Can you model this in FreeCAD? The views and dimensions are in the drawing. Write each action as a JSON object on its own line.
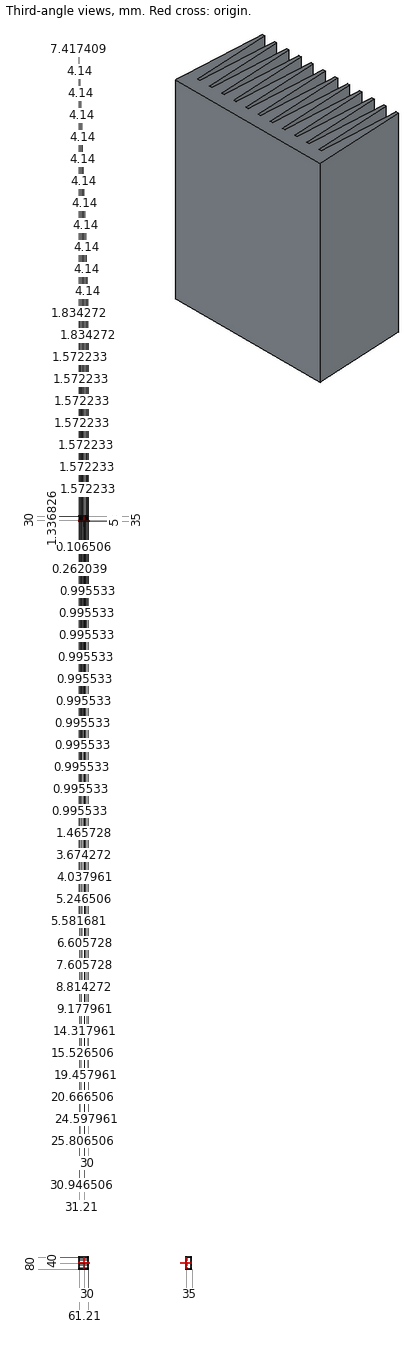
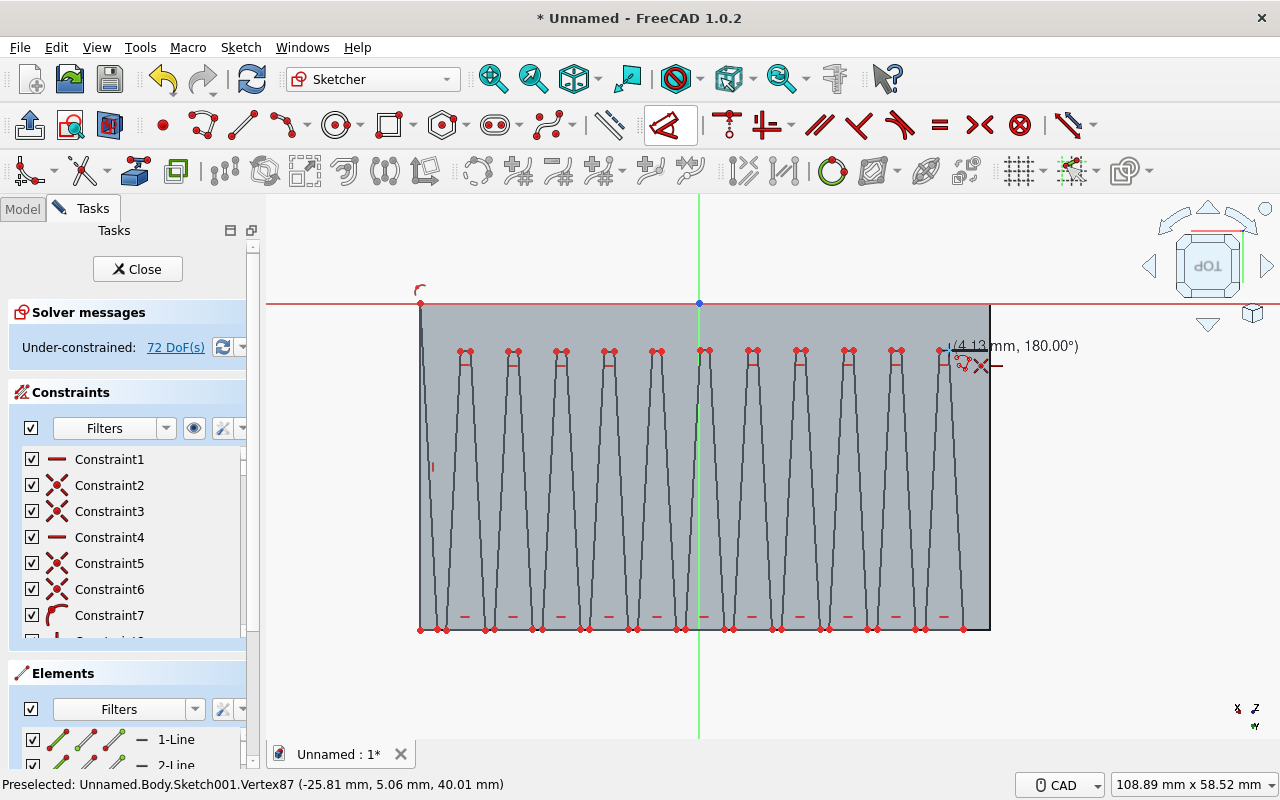
{"action": "scroll", "coordinate": [973, 630], "scroll_direction": "up", "scroll_amount": 3}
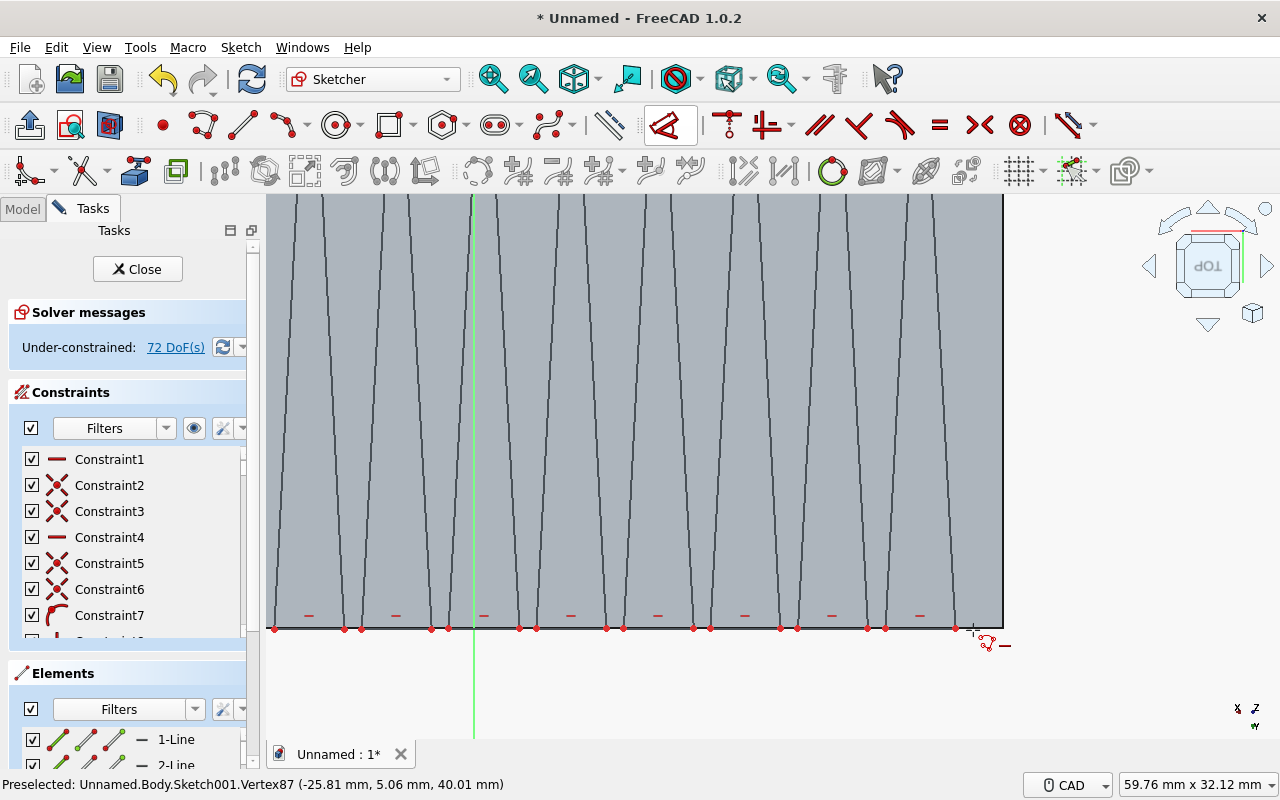
{"action": "left_click", "coordinate": [972, 628]}
{"action": "left_click", "coordinate": [1003, 628]}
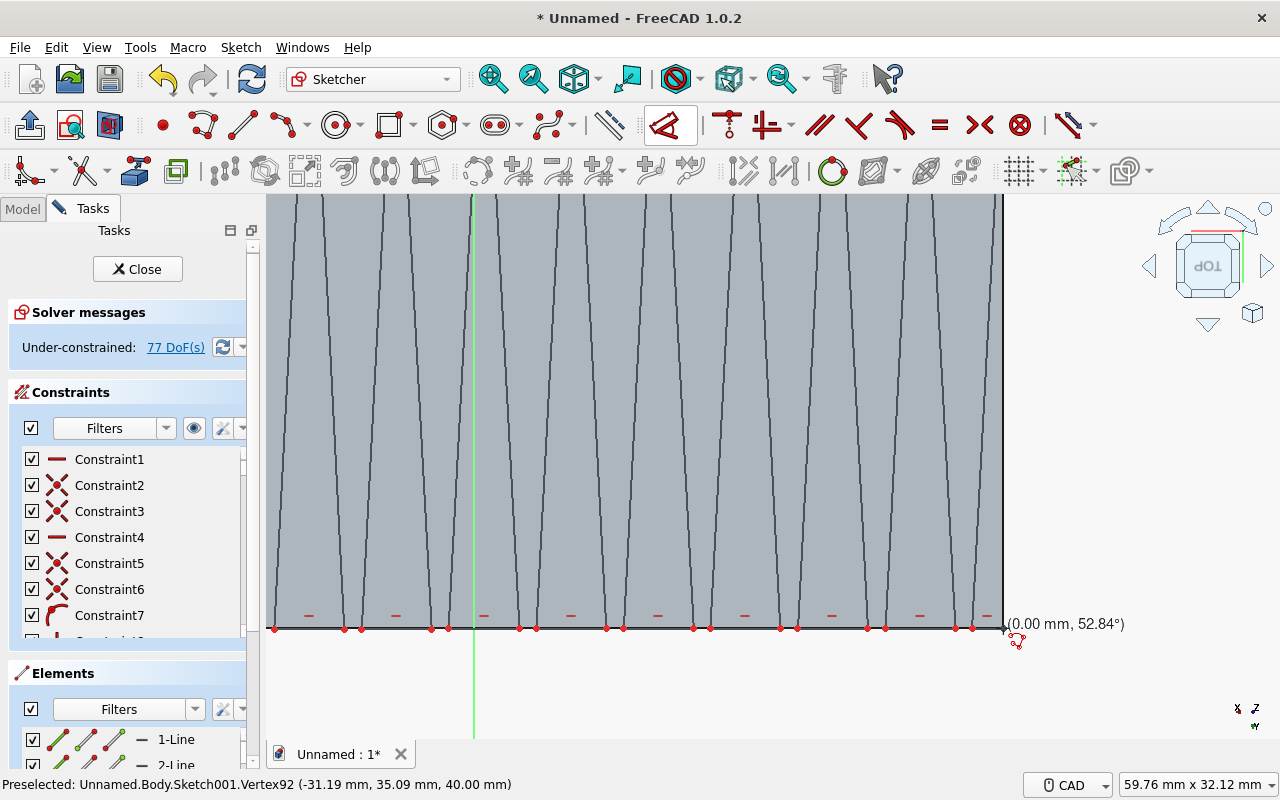
{"action": "scroll", "coordinate": [973, 631], "scroll_direction": "down", "scroll_amount": 3}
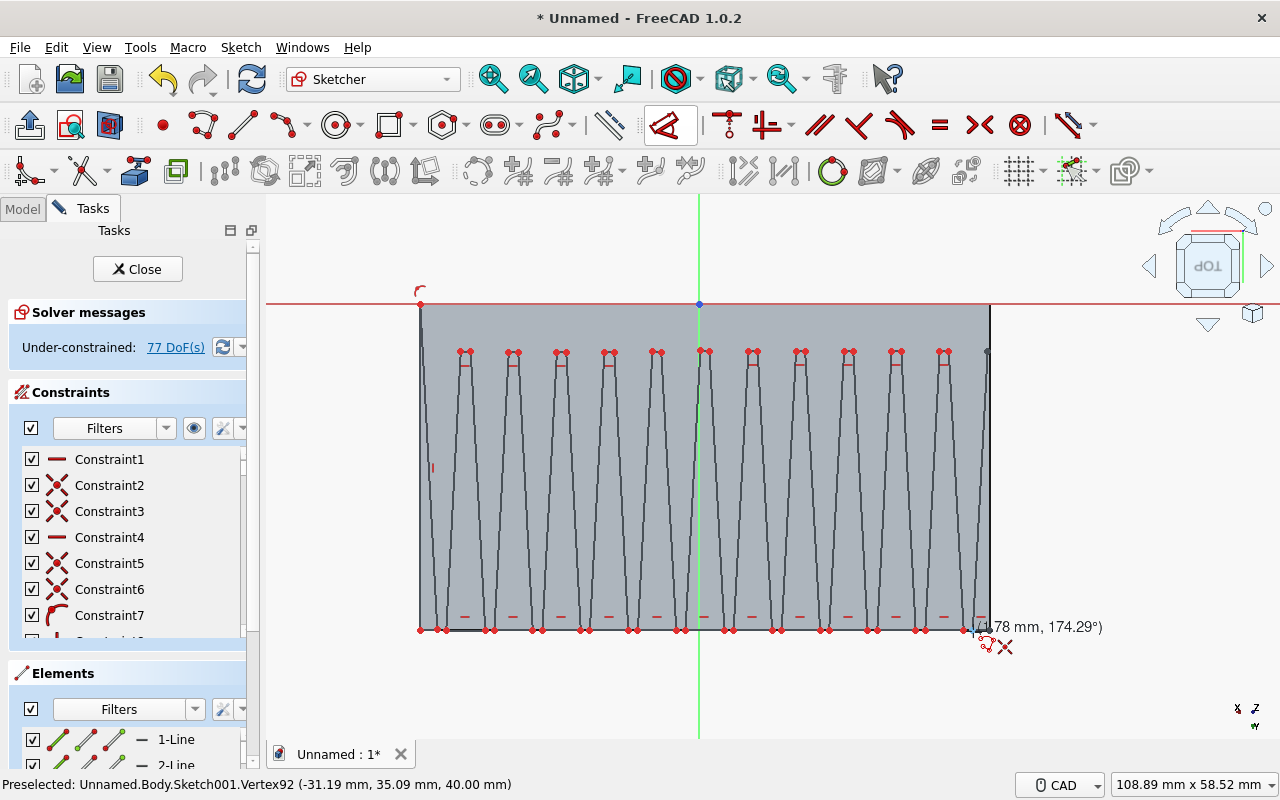
{"action": "scroll", "coordinate": [990, 351], "scroll_direction": "up", "scroll_amount": 10}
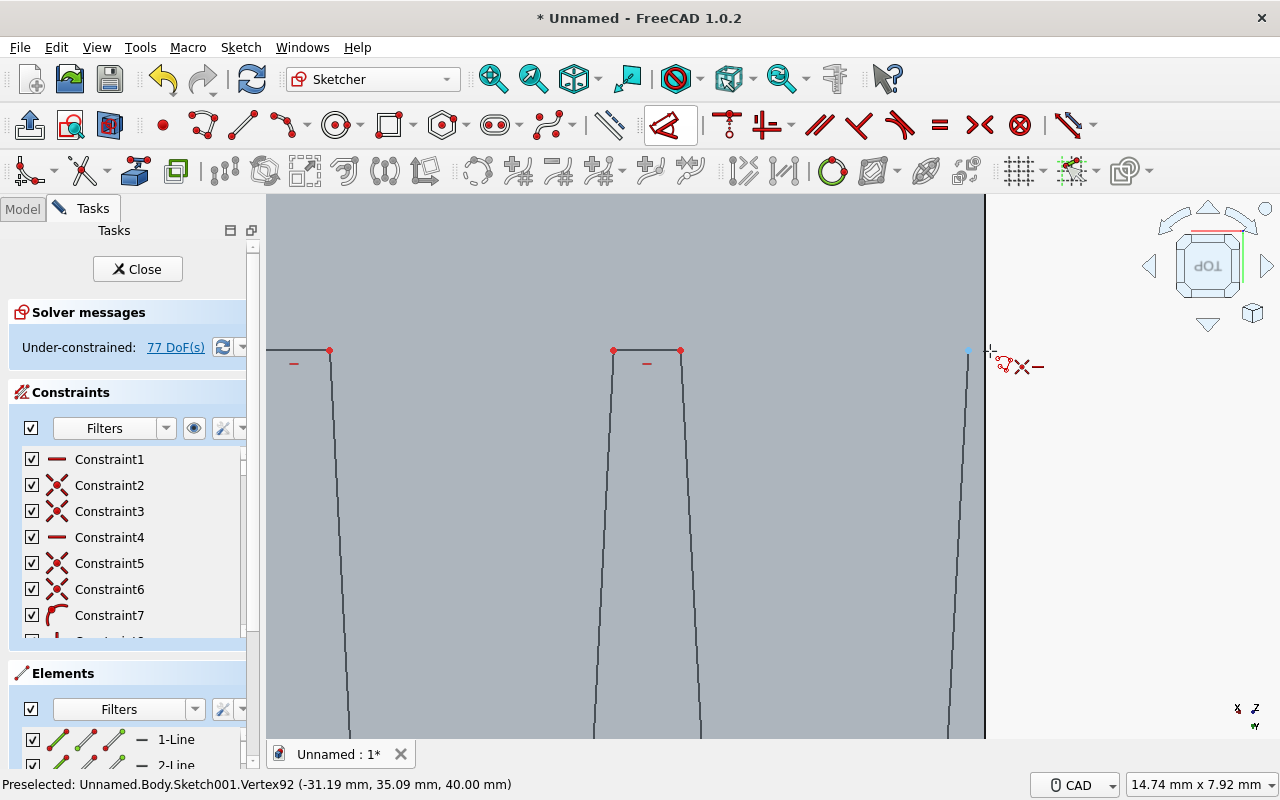
{"action": "left_click", "coordinate": [984, 346]}
{"action": "left_click", "coordinate": [969, 350]}
{"action": "key", "text": "Escape"}
{"action": "key", "text": "Escape"}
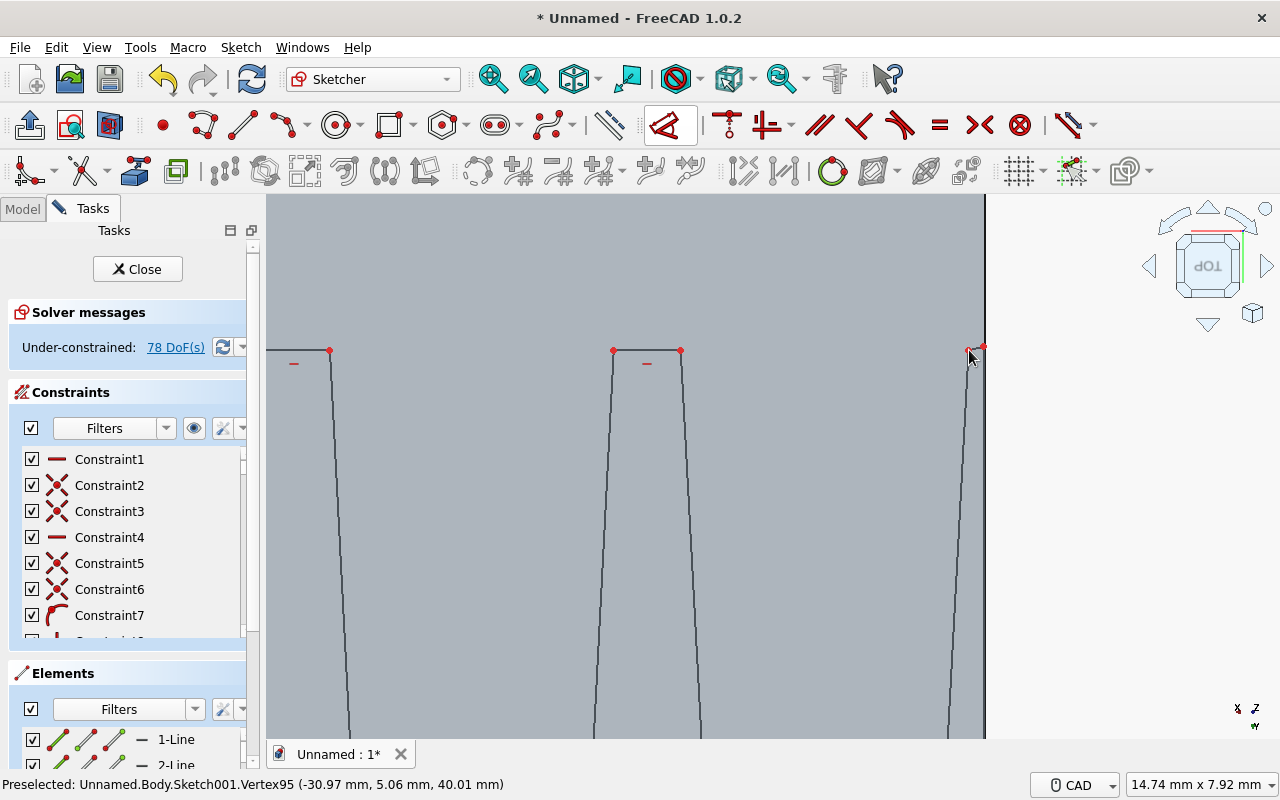
{"action": "scroll", "coordinate": [990, 351], "scroll_direction": "down", "scroll_amount": 10}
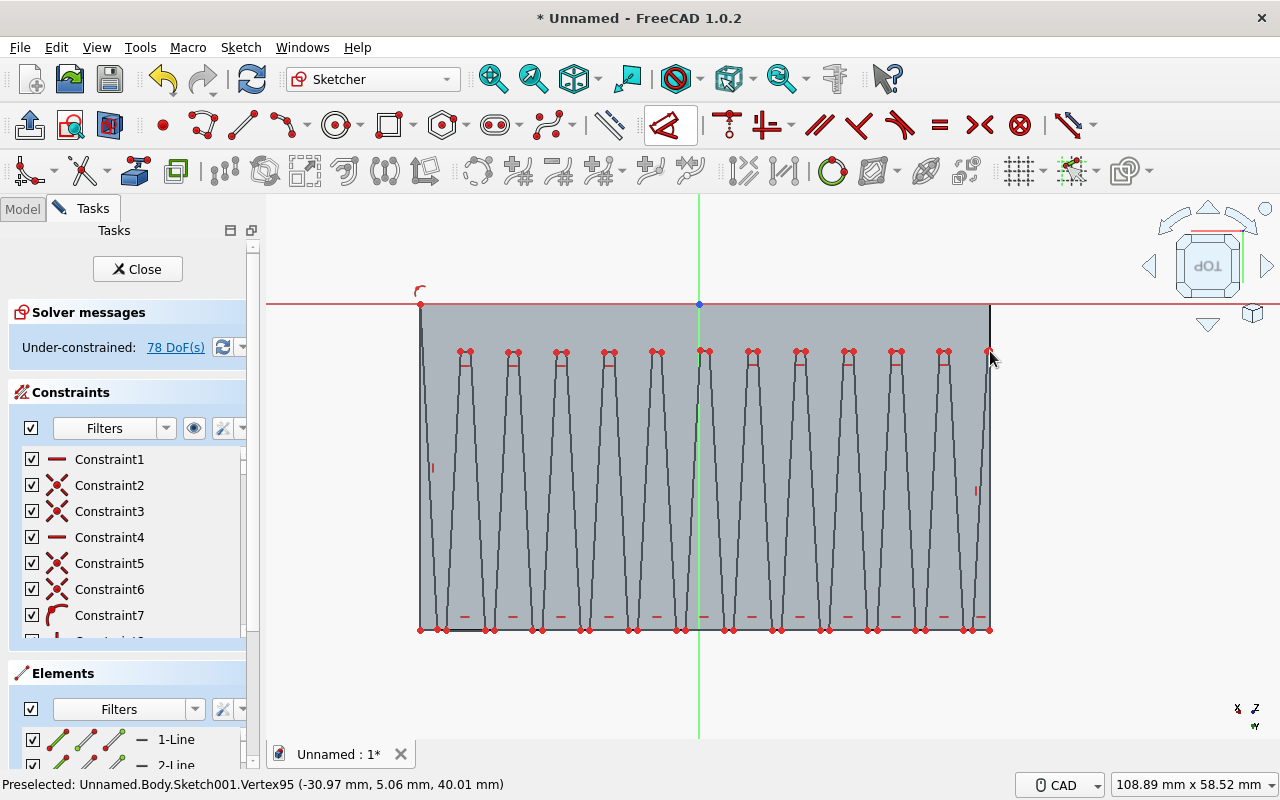
{"action": "scroll", "coordinate": [425, 630], "scroll_direction": "up", "scroll_amount": 5}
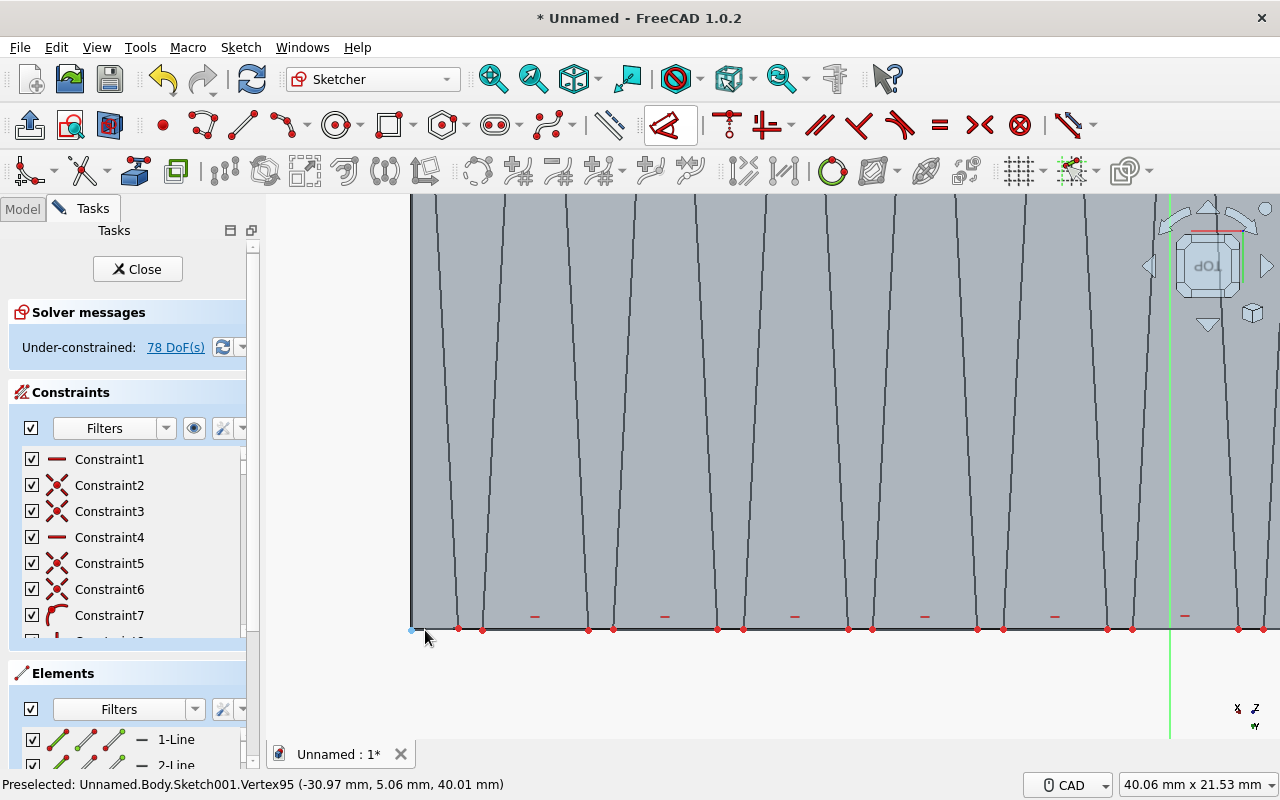
{"action": "left_click", "coordinate": [426, 630]}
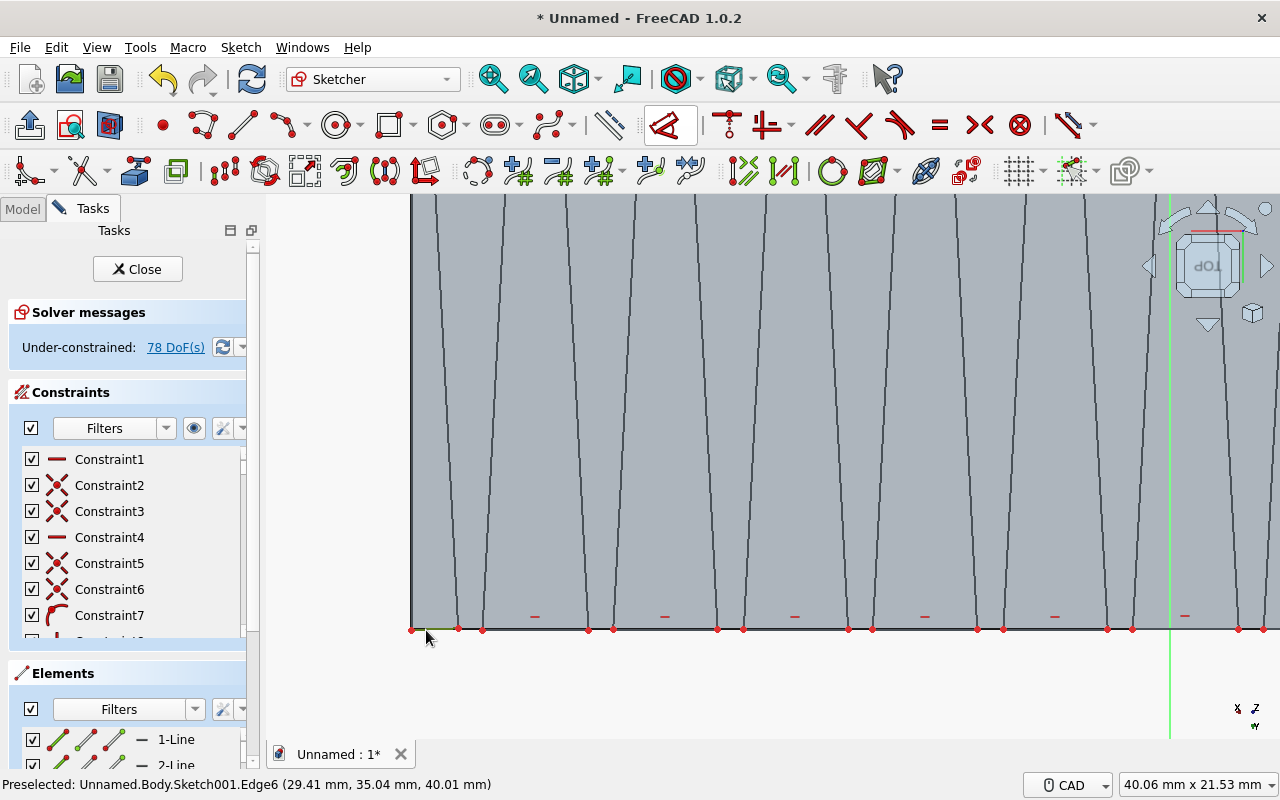
{"action": "left_click", "coordinate": [794, 126]}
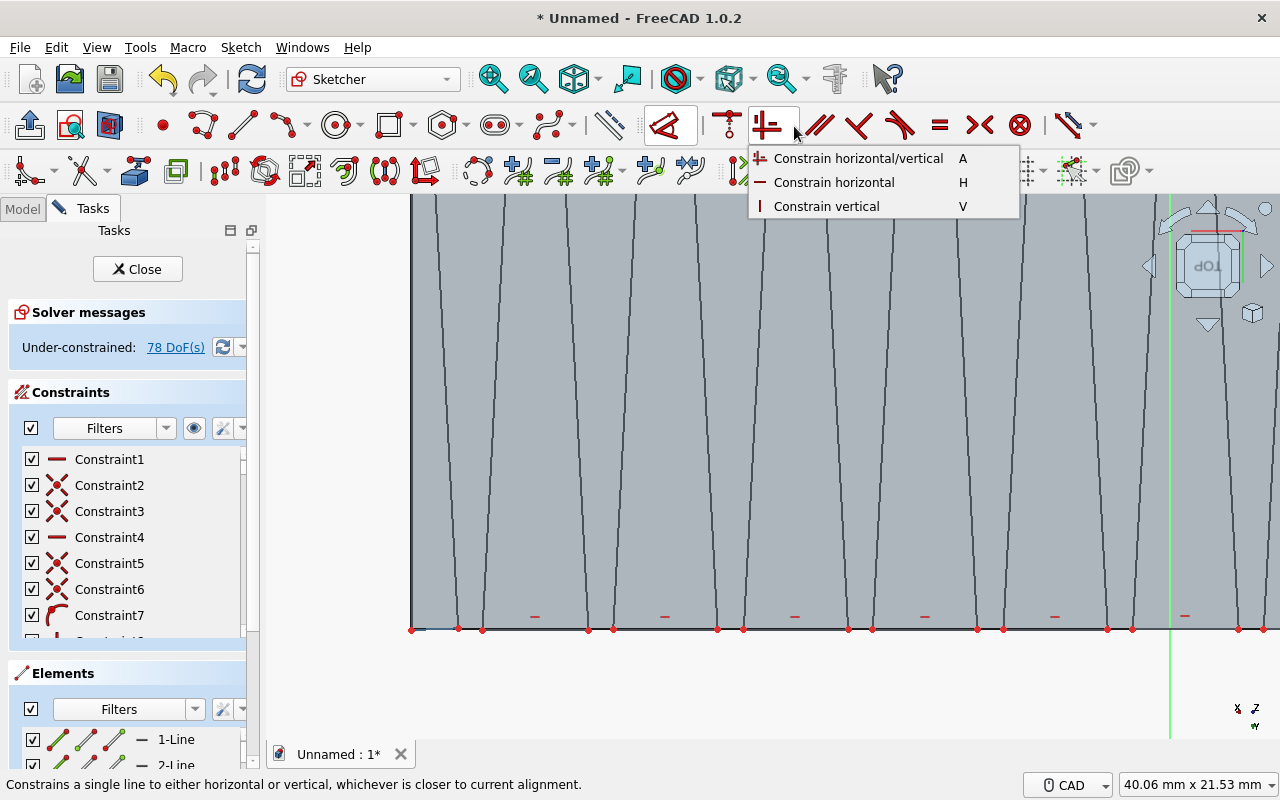
{"action": "left_click", "coordinate": [884, 182]}